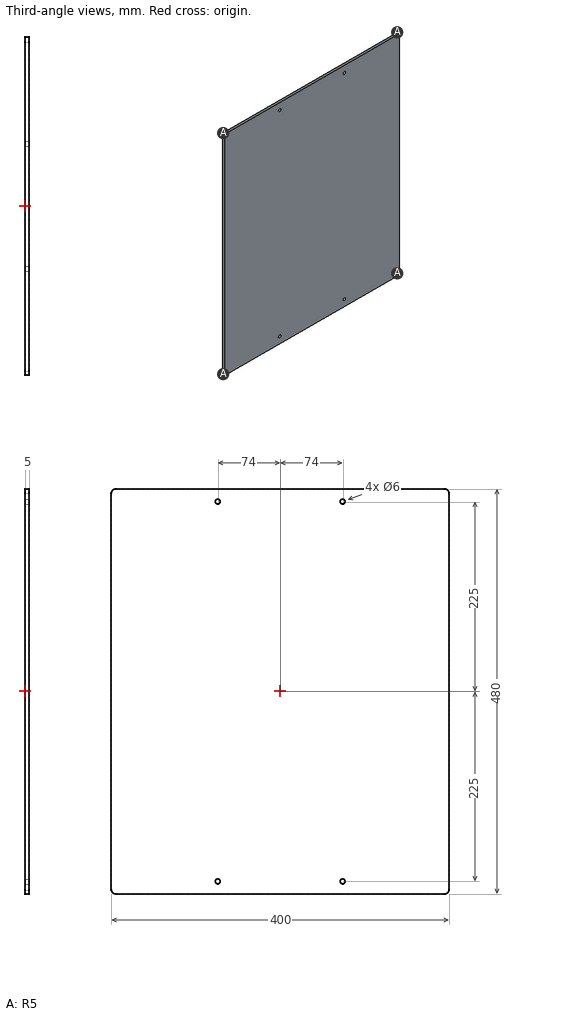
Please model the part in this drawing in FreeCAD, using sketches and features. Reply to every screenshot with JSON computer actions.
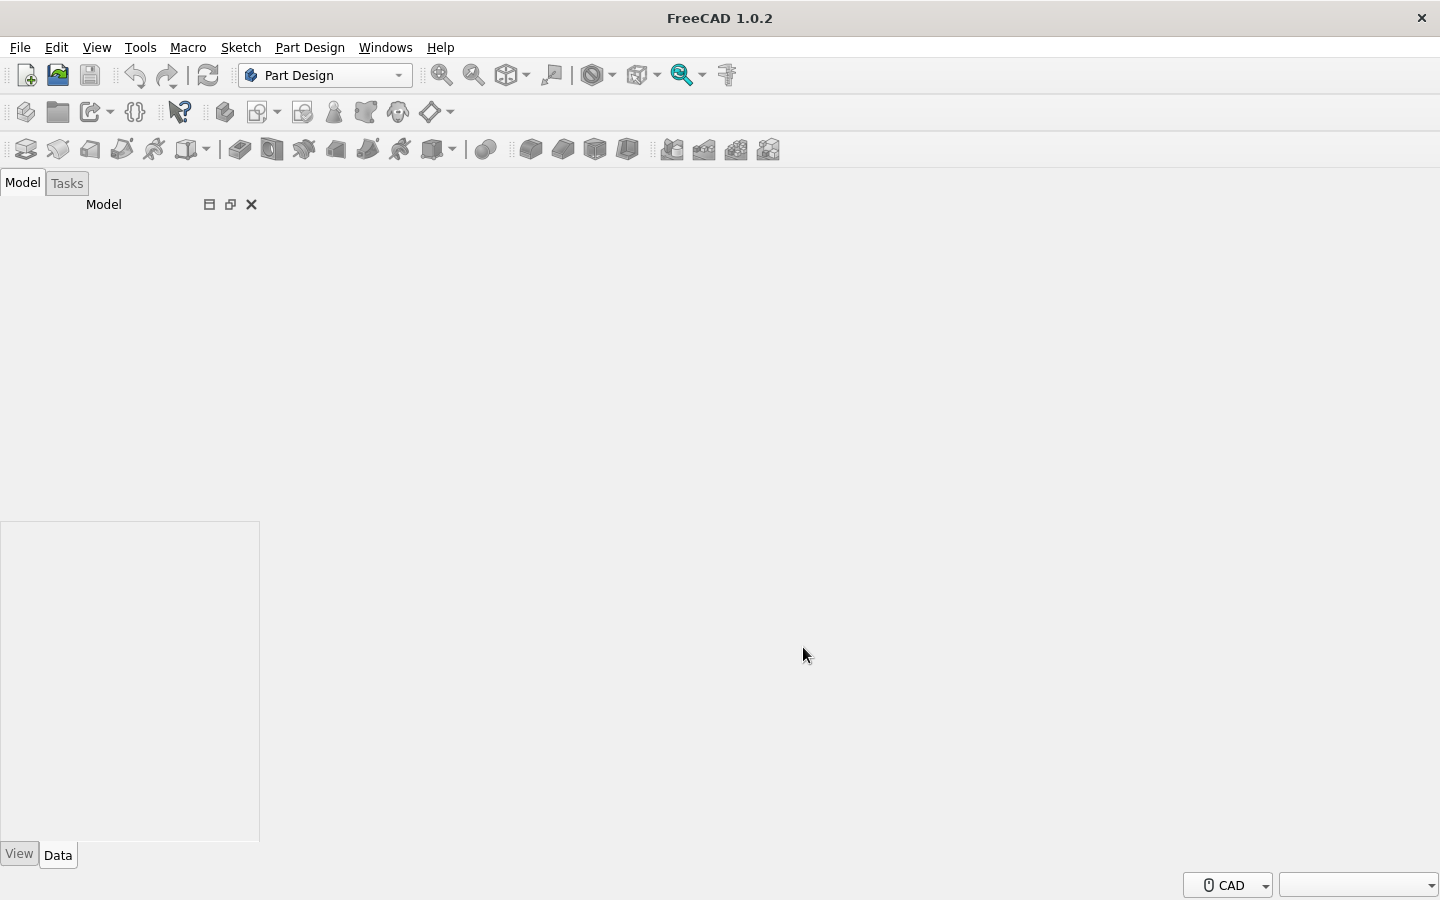
{"action": "left_click", "coordinate": [26, 76]}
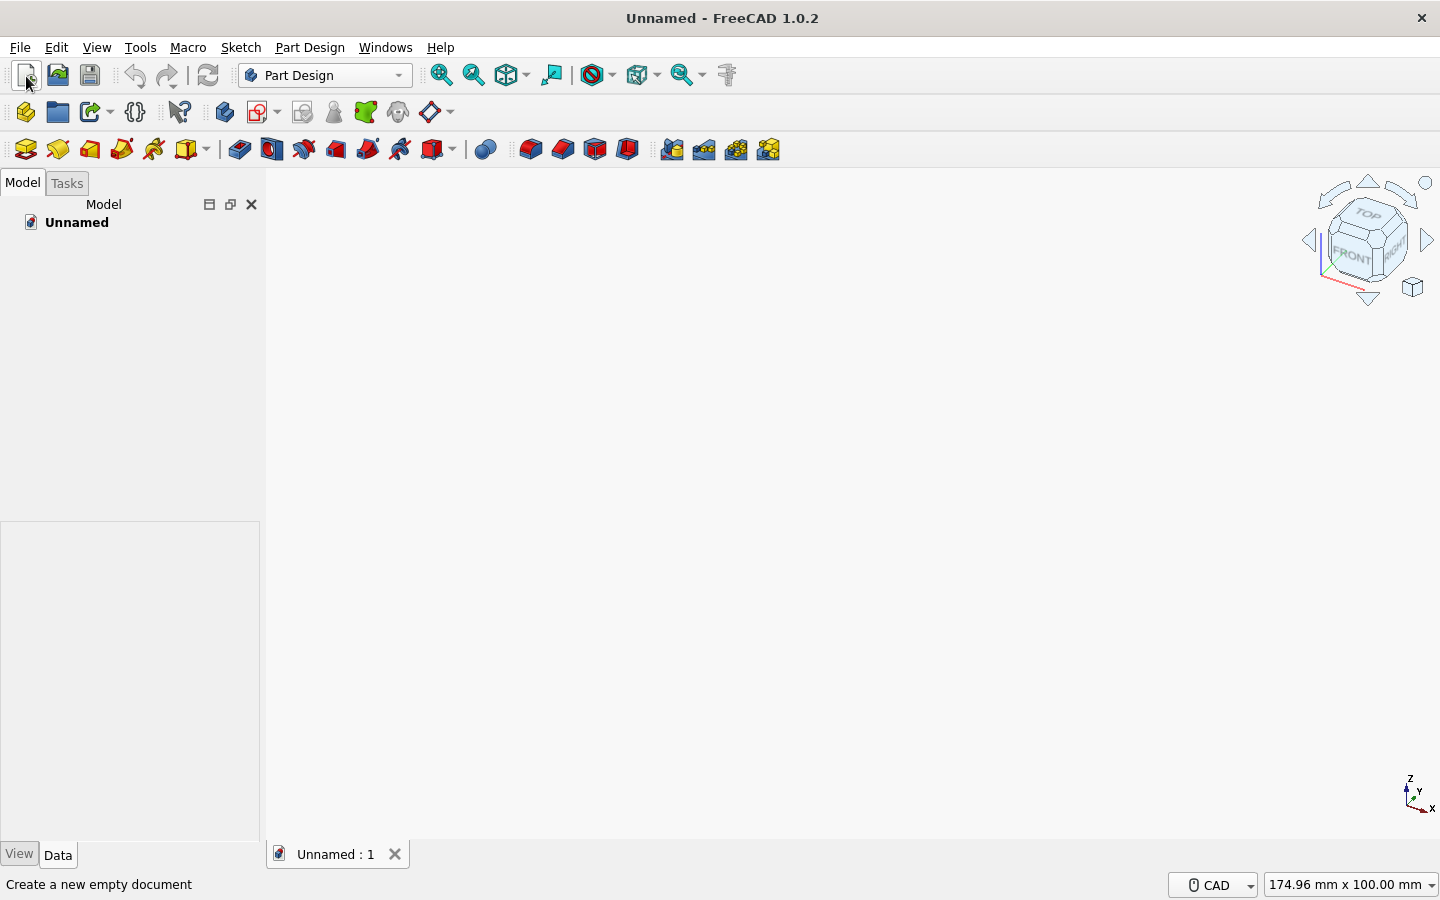
{"action": "left_click", "coordinate": [258, 112]}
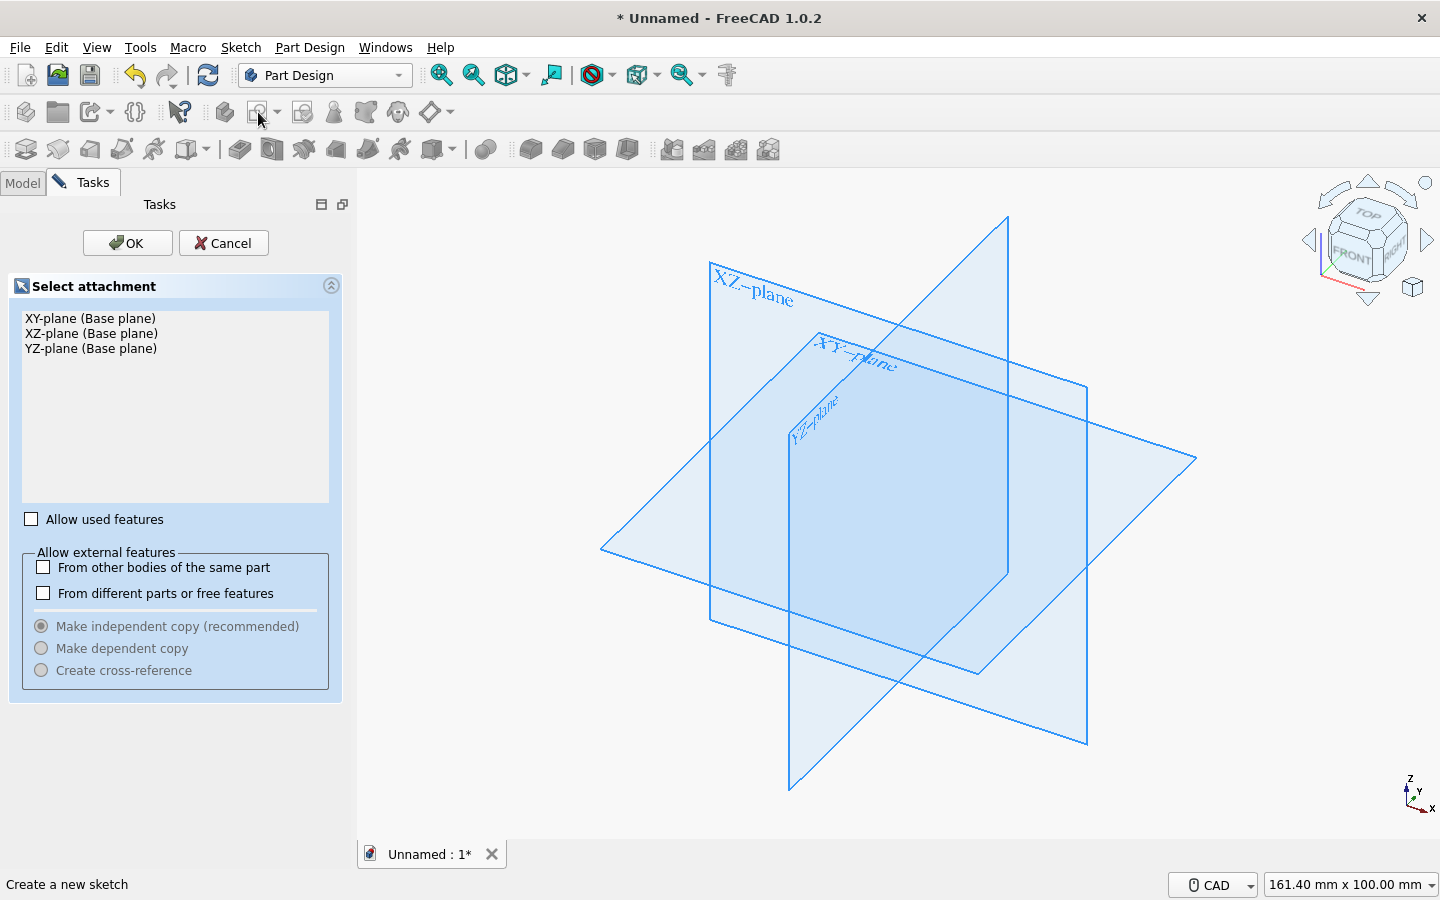
{"action": "left_click", "coordinate": [82, 348]}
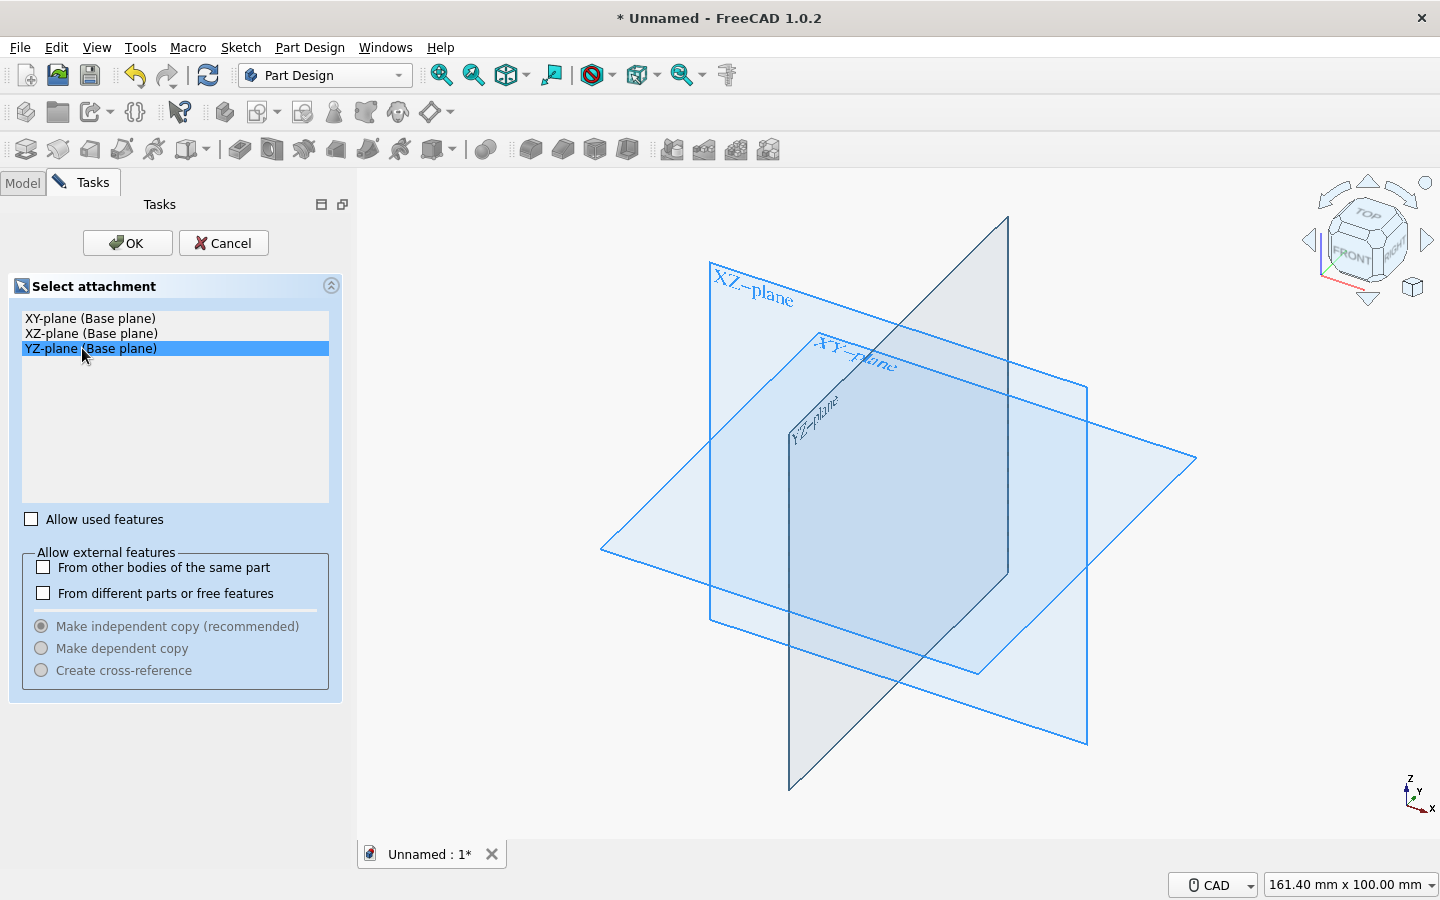
{"action": "left_click", "coordinate": [128, 243]}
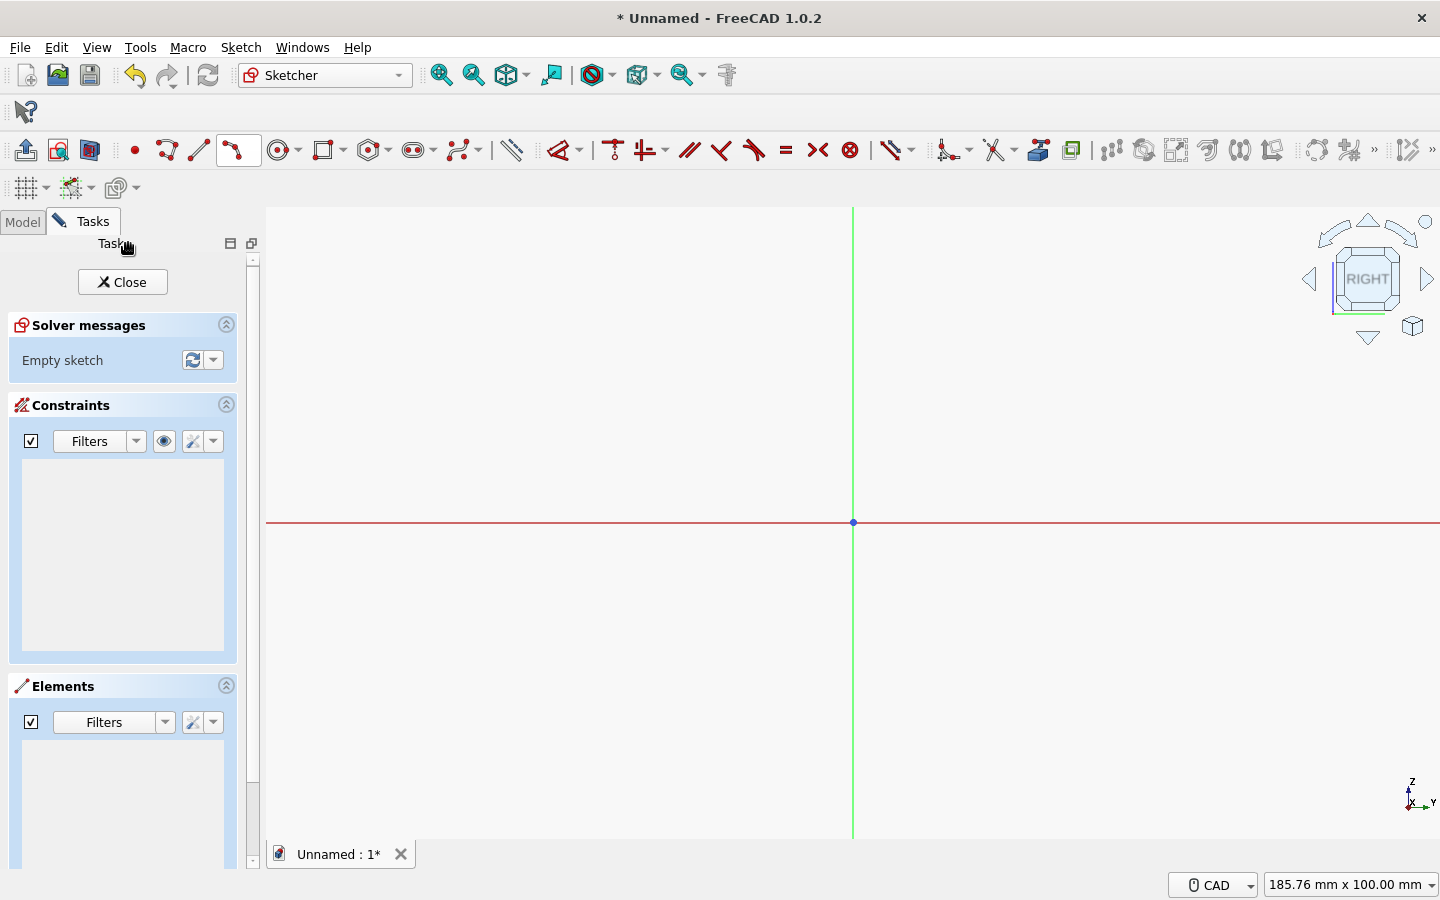
{"action": "scroll", "coordinate": [774, 523], "scroll_direction": "down", "scroll_amount": 10}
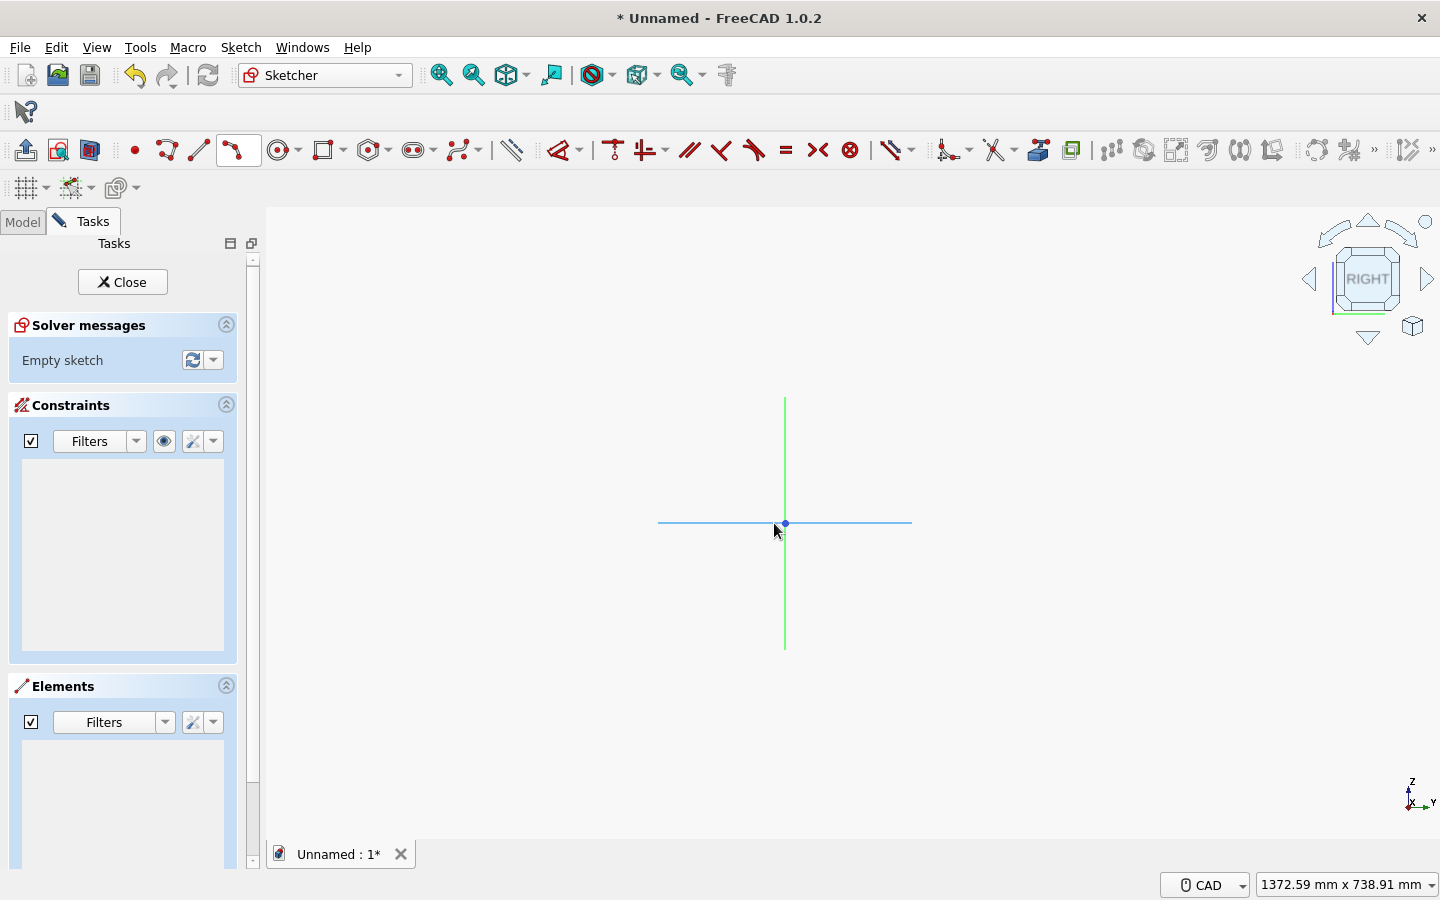
{"action": "key", "text": "g v"}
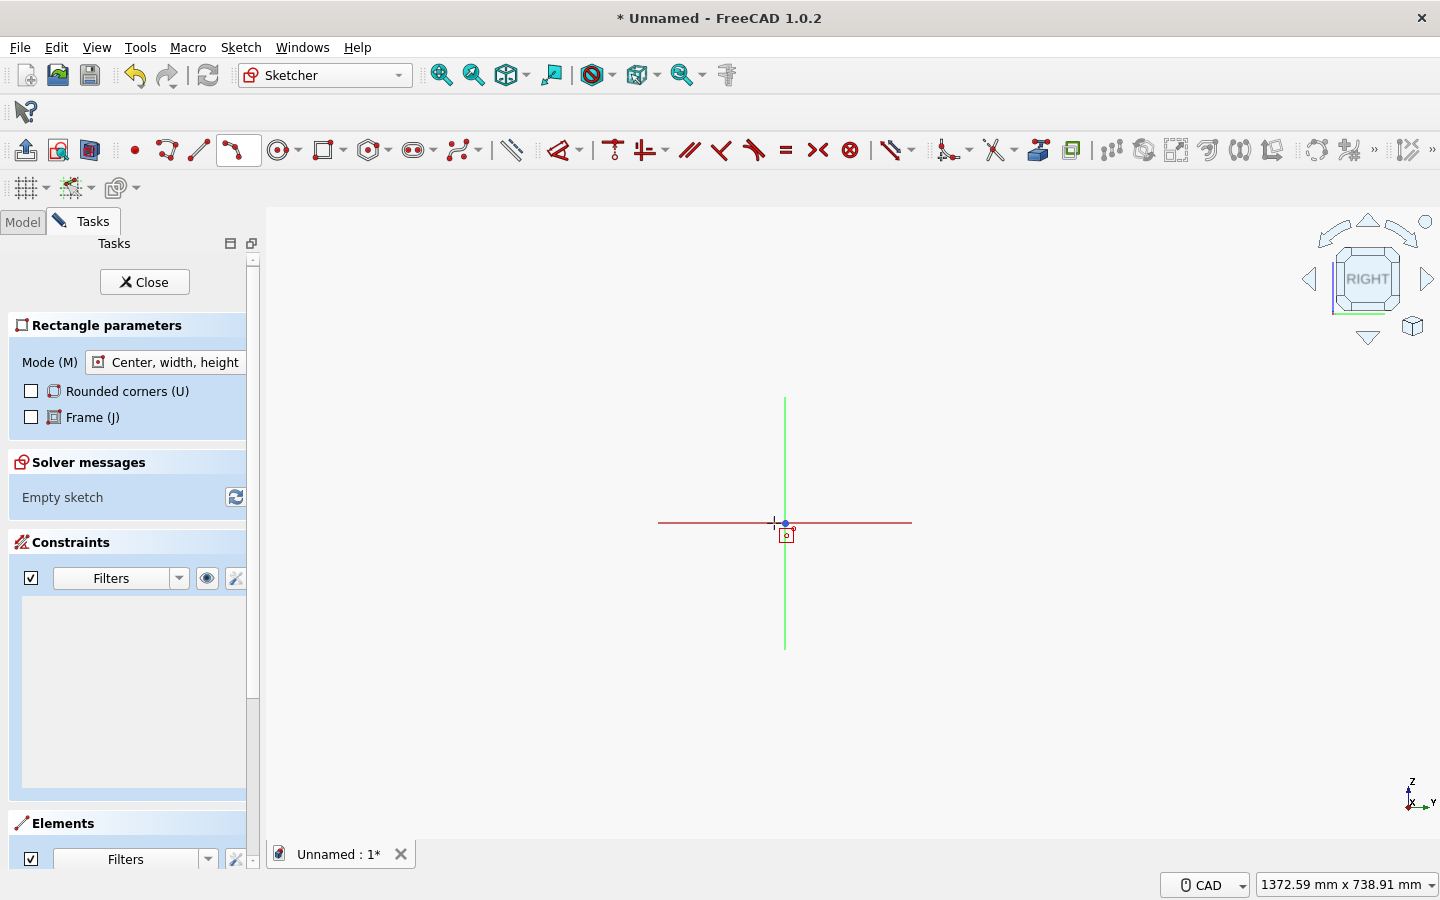
{"action": "left_click", "coordinate": [785, 523]}
{"action": "left_click", "coordinate": [956, 318]}
{"action": "key", "text": "Escape"}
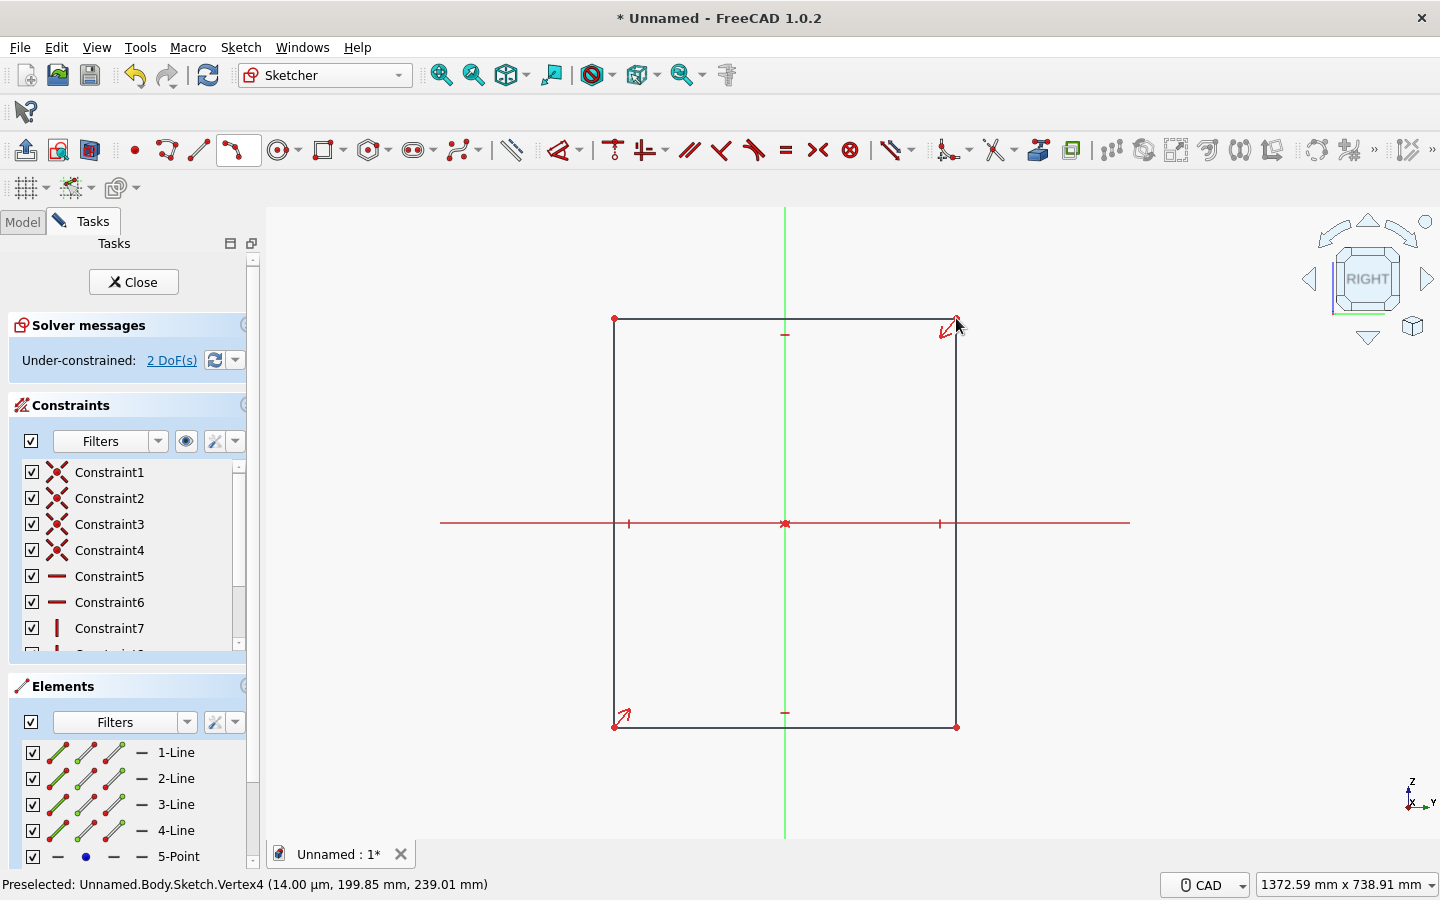
{"action": "left_click", "coordinate": [558, 150]}